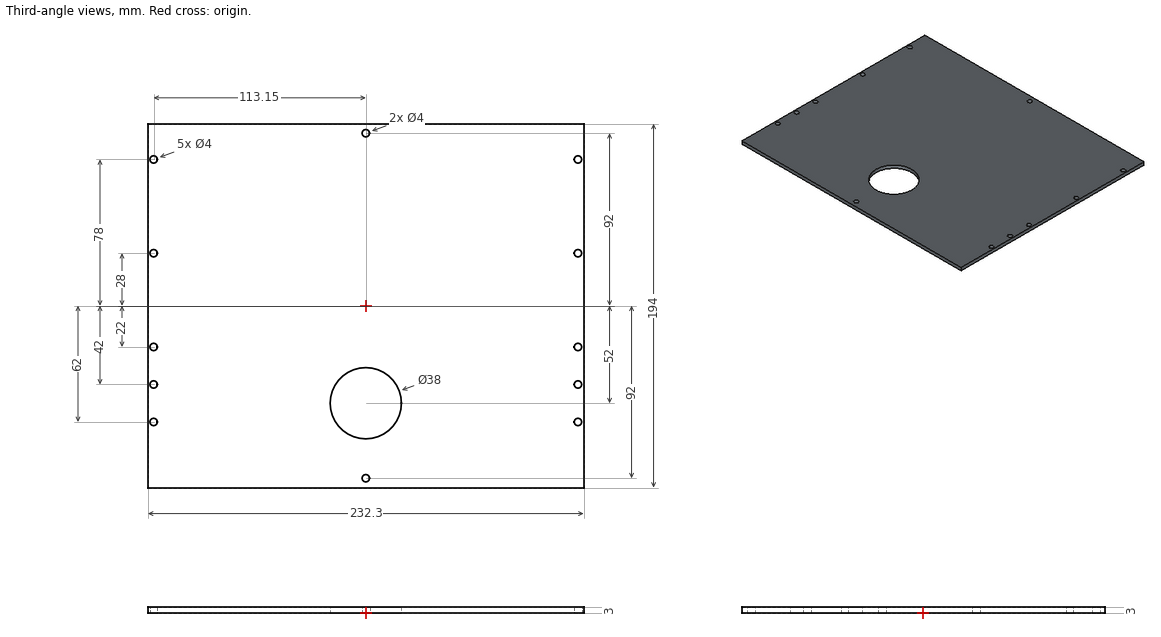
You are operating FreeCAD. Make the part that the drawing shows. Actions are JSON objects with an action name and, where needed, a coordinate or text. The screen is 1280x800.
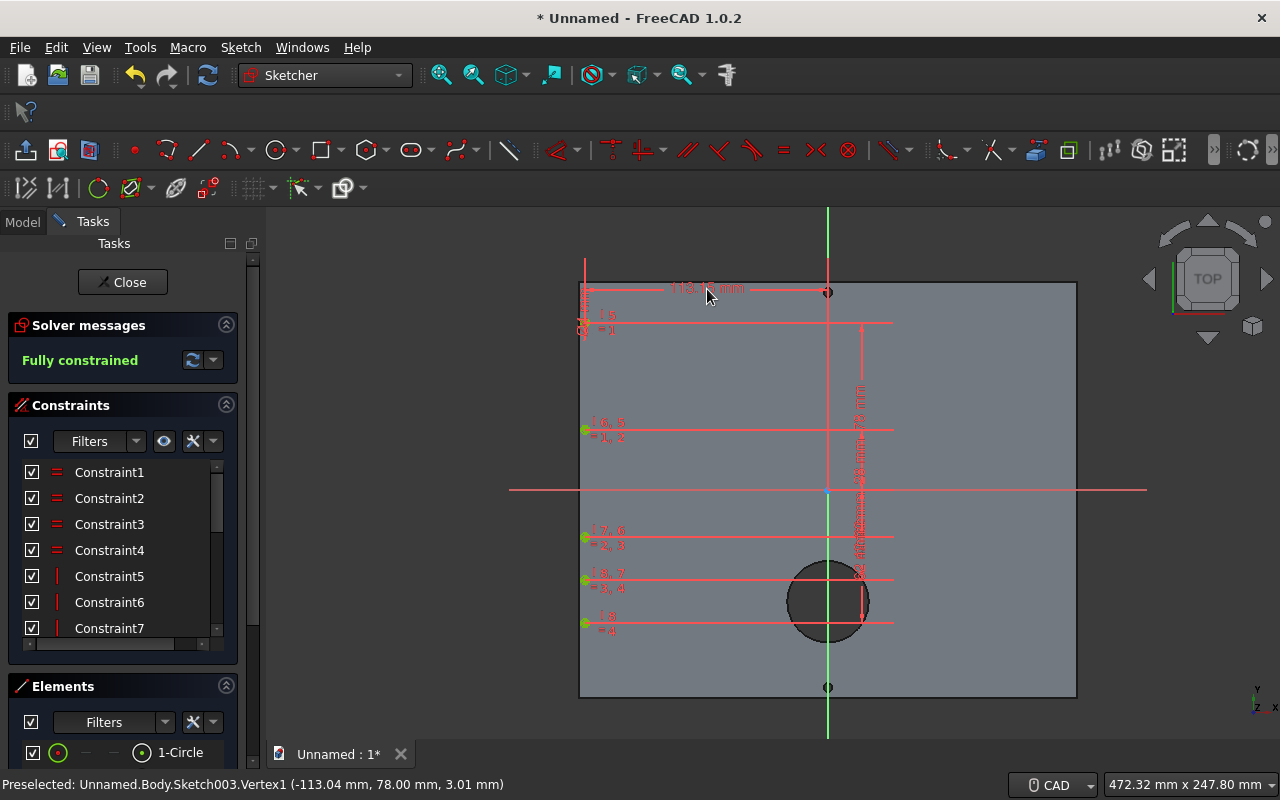
{"action": "left_click", "coordinate": [123, 282]}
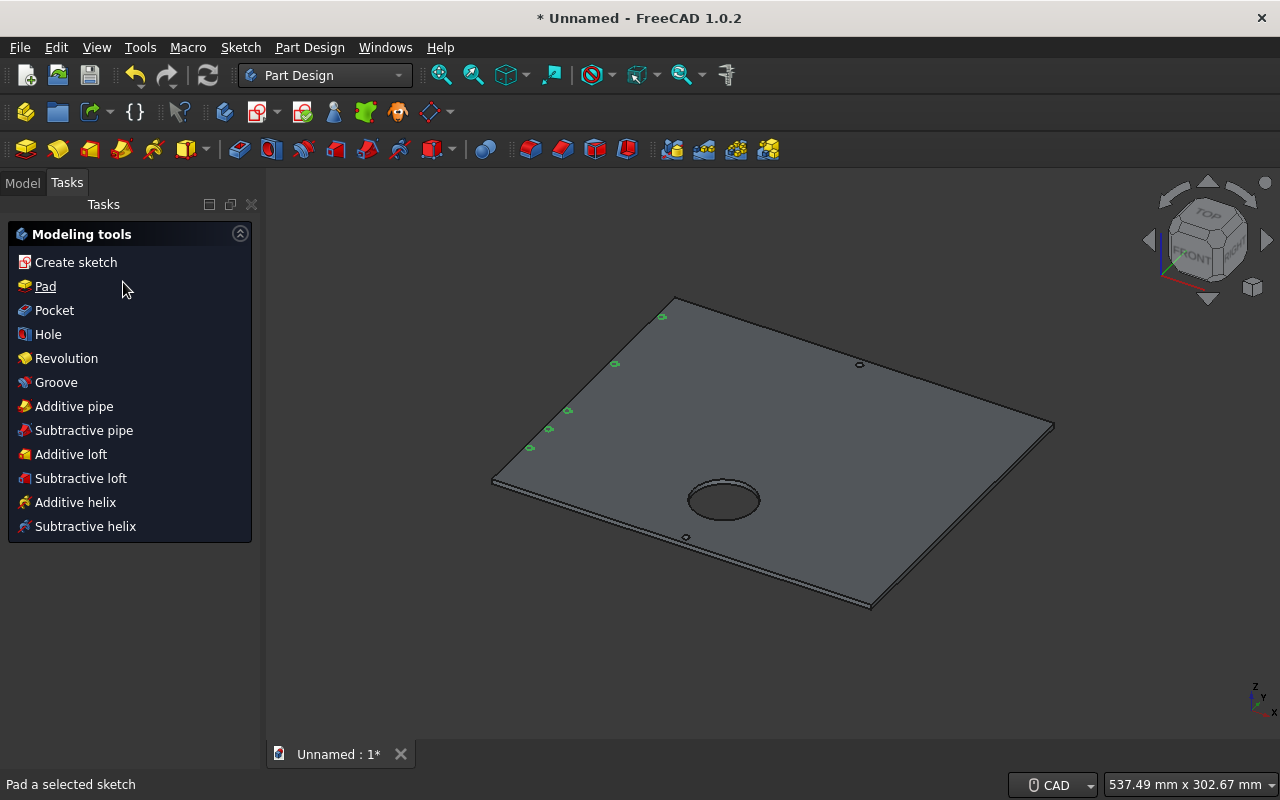
{"action": "left_click", "coordinate": [240, 150]}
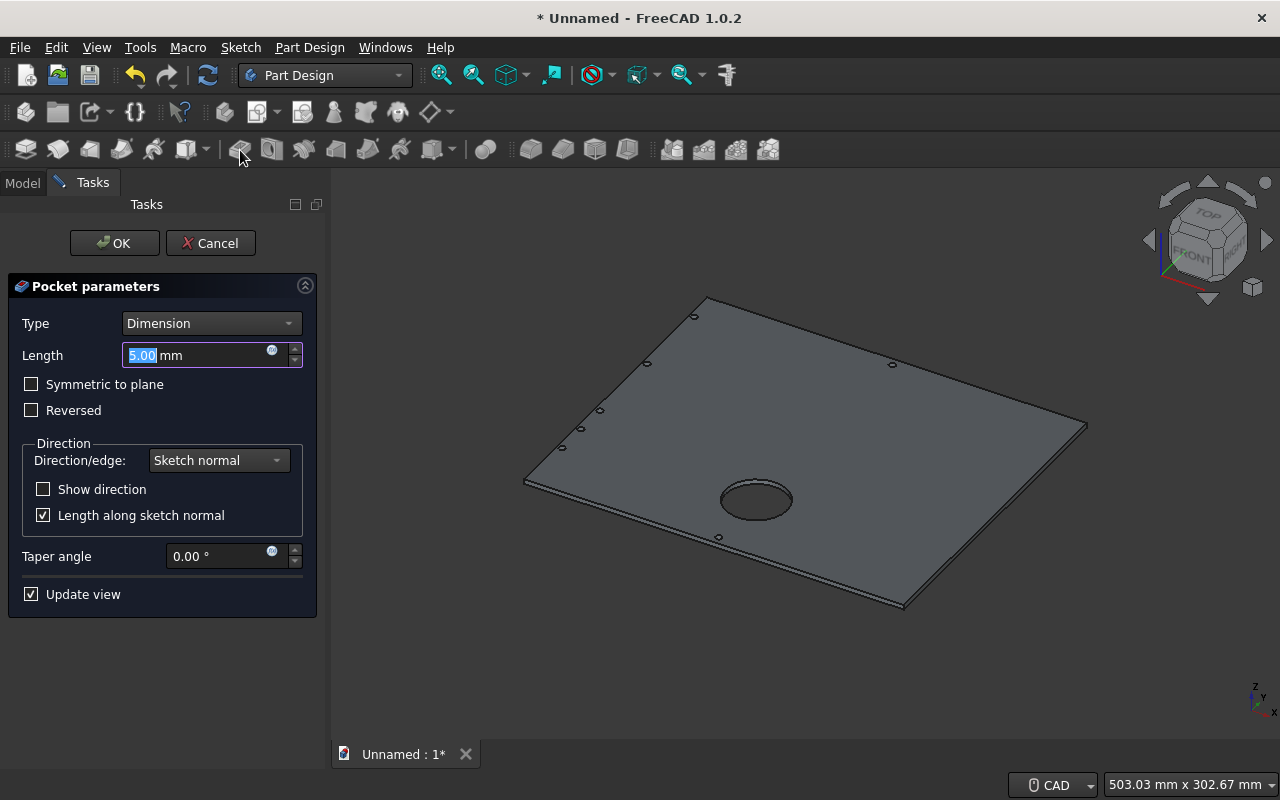
{"action": "left_click", "coordinate": [212, 324]}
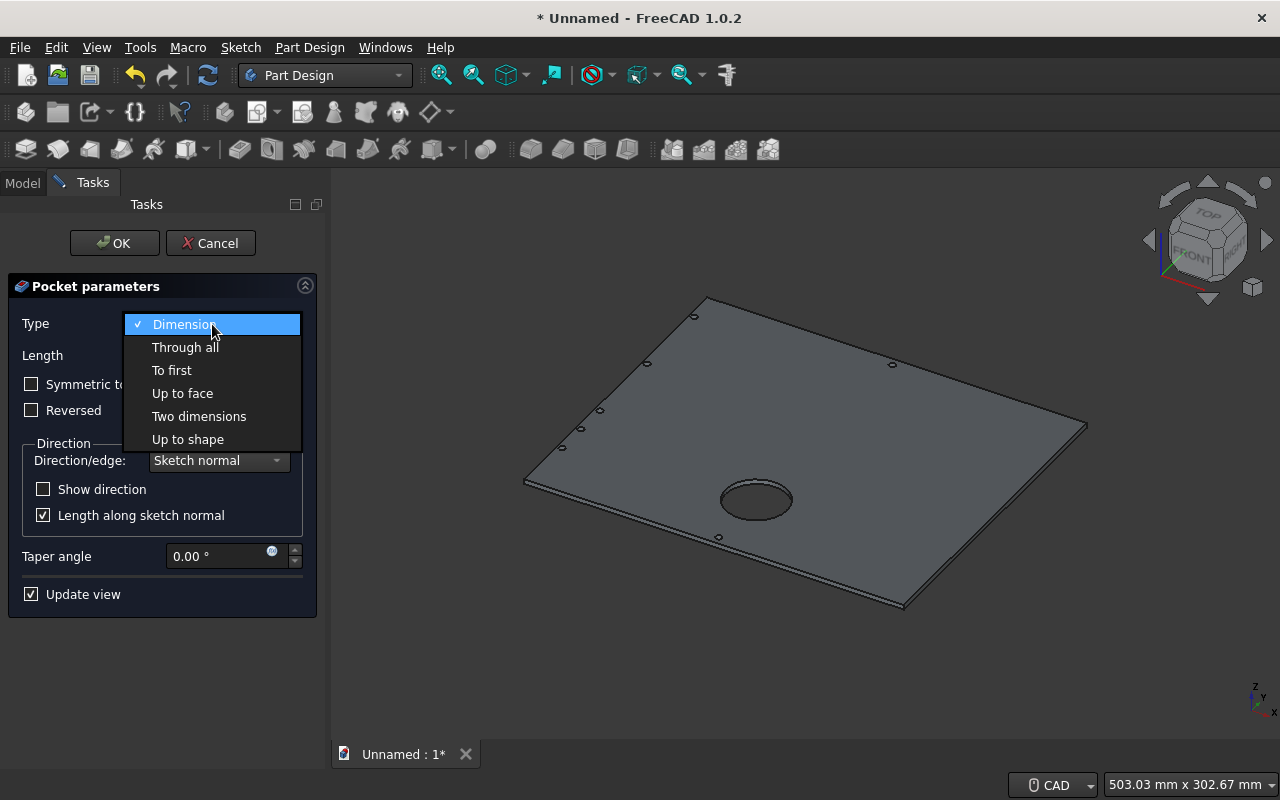
{"action": "left_click", "coordinate": [212, 348]}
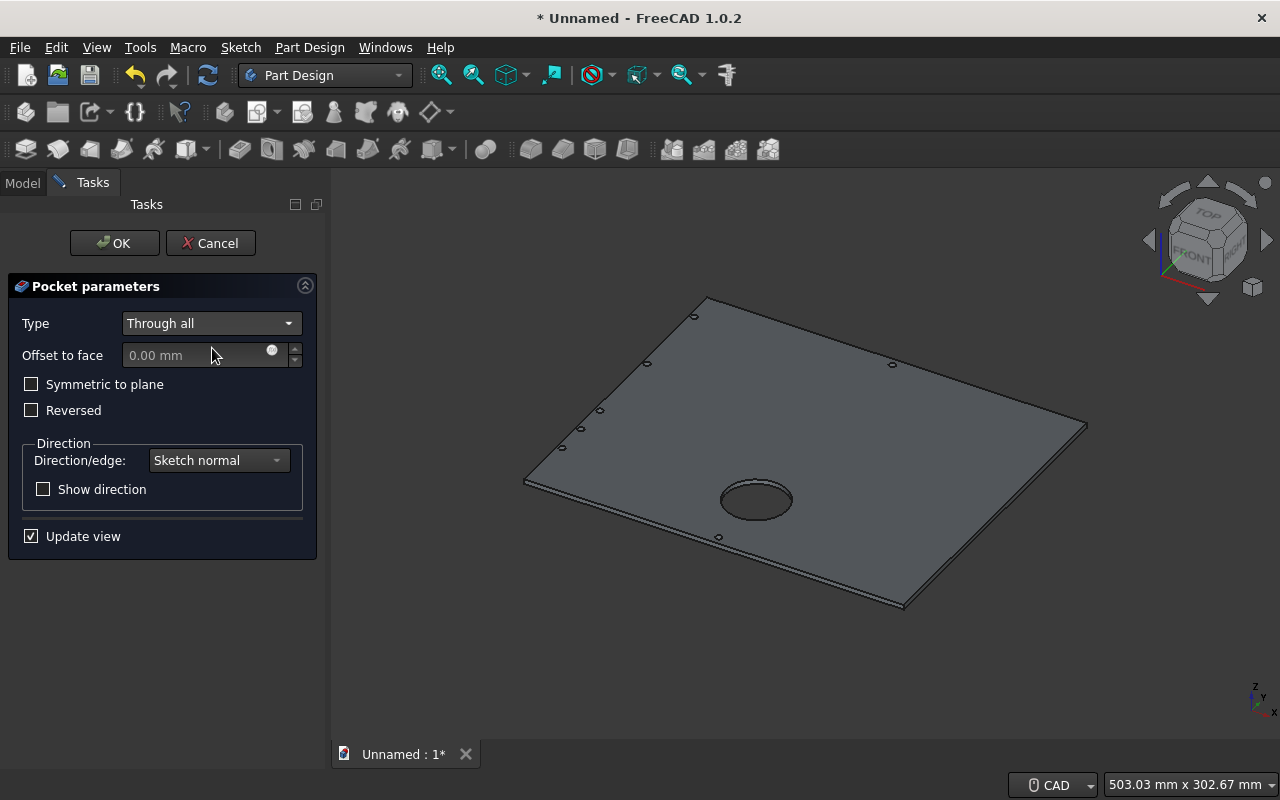
{"action": "left_click", "coordinate": [115, 243]}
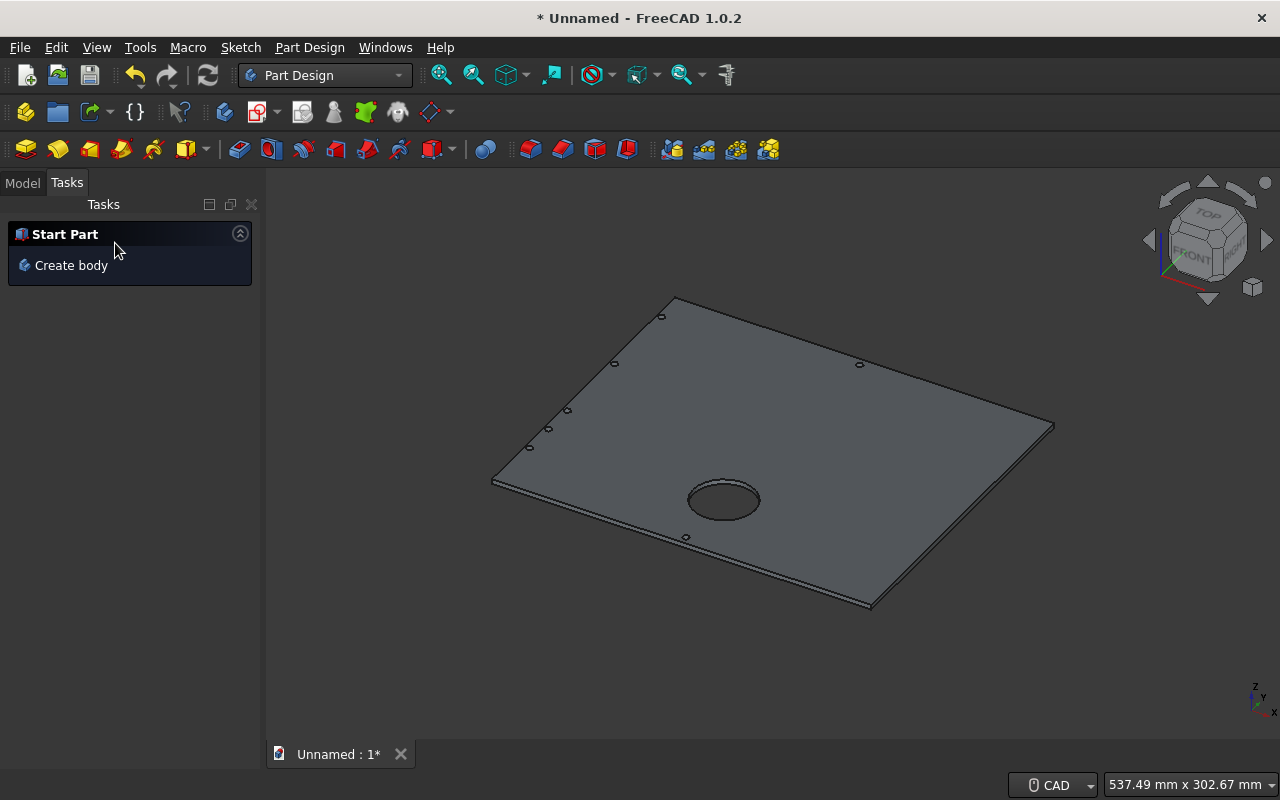
{"action": "left_click", "coordinate": [23, 182]}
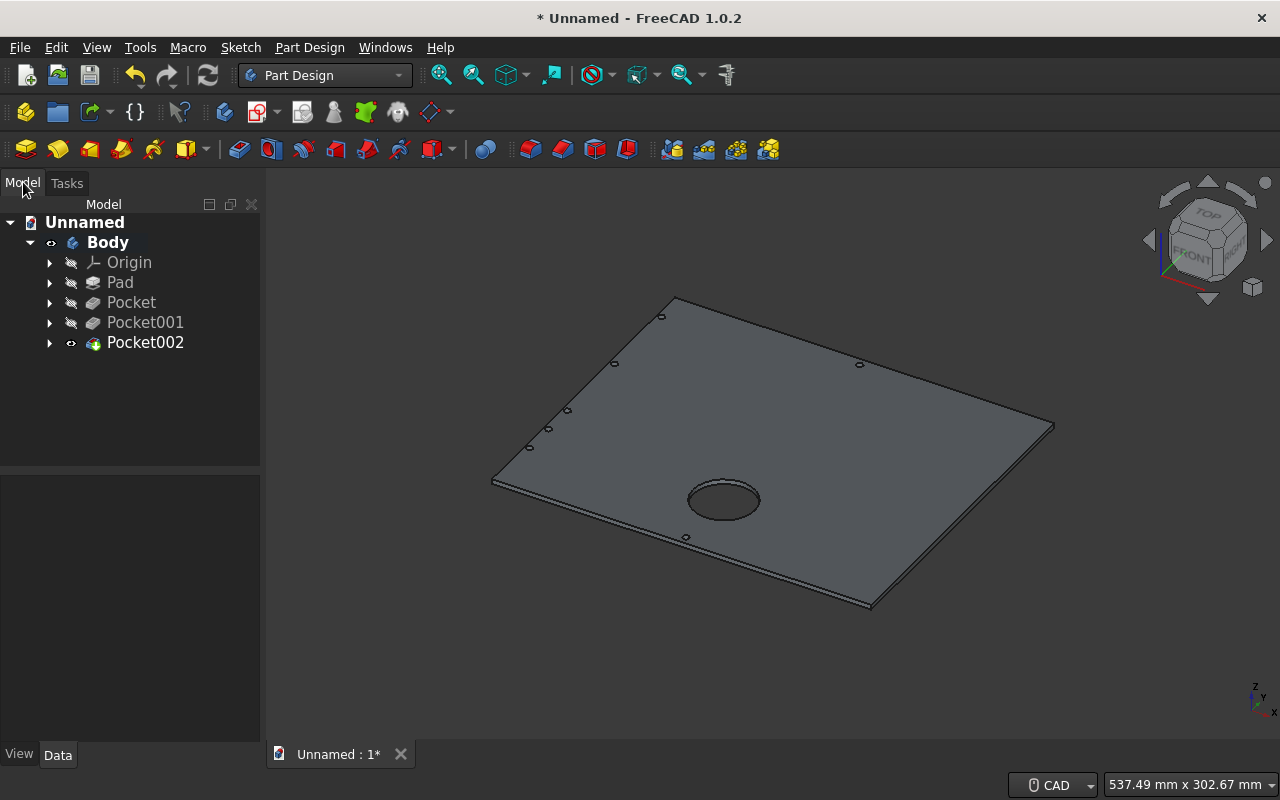
{"action": "left_click", "coordinate": [116, 343]}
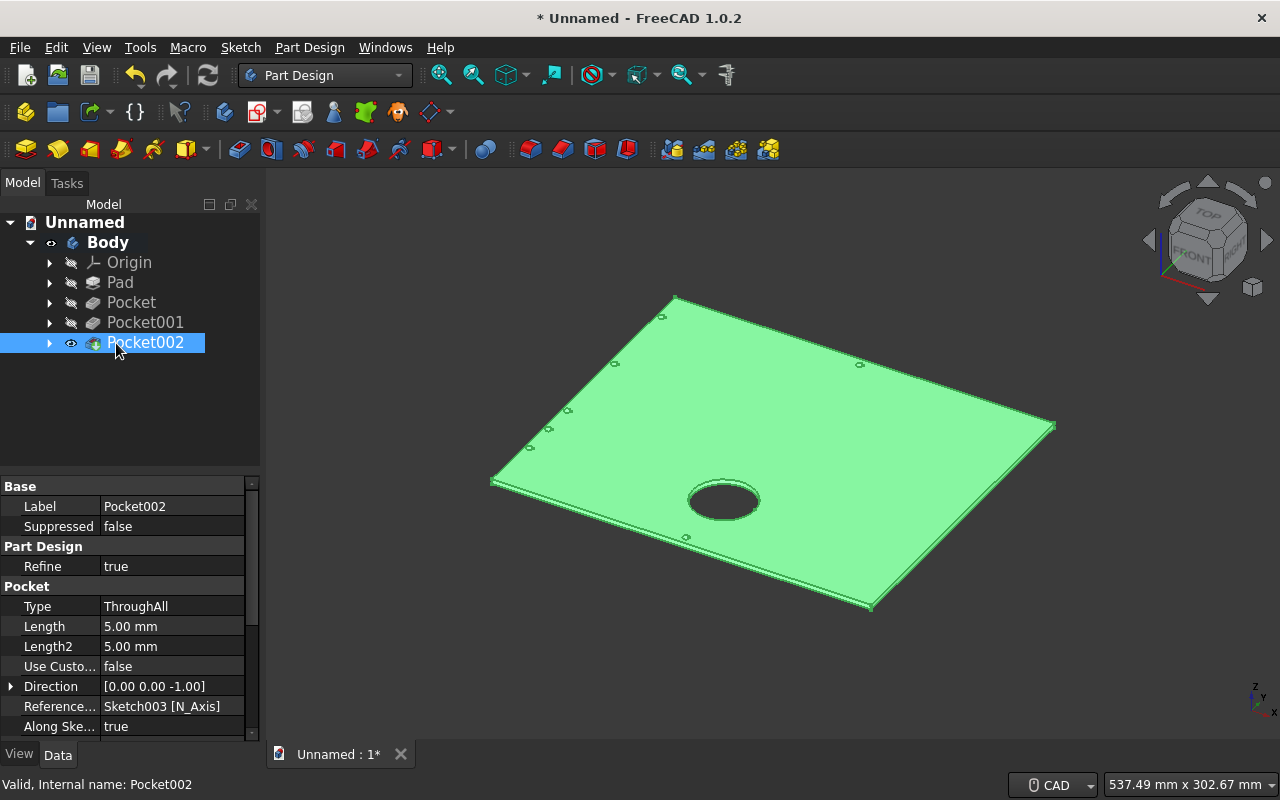
{"action": "left_click", "coordinate": [672, 150]}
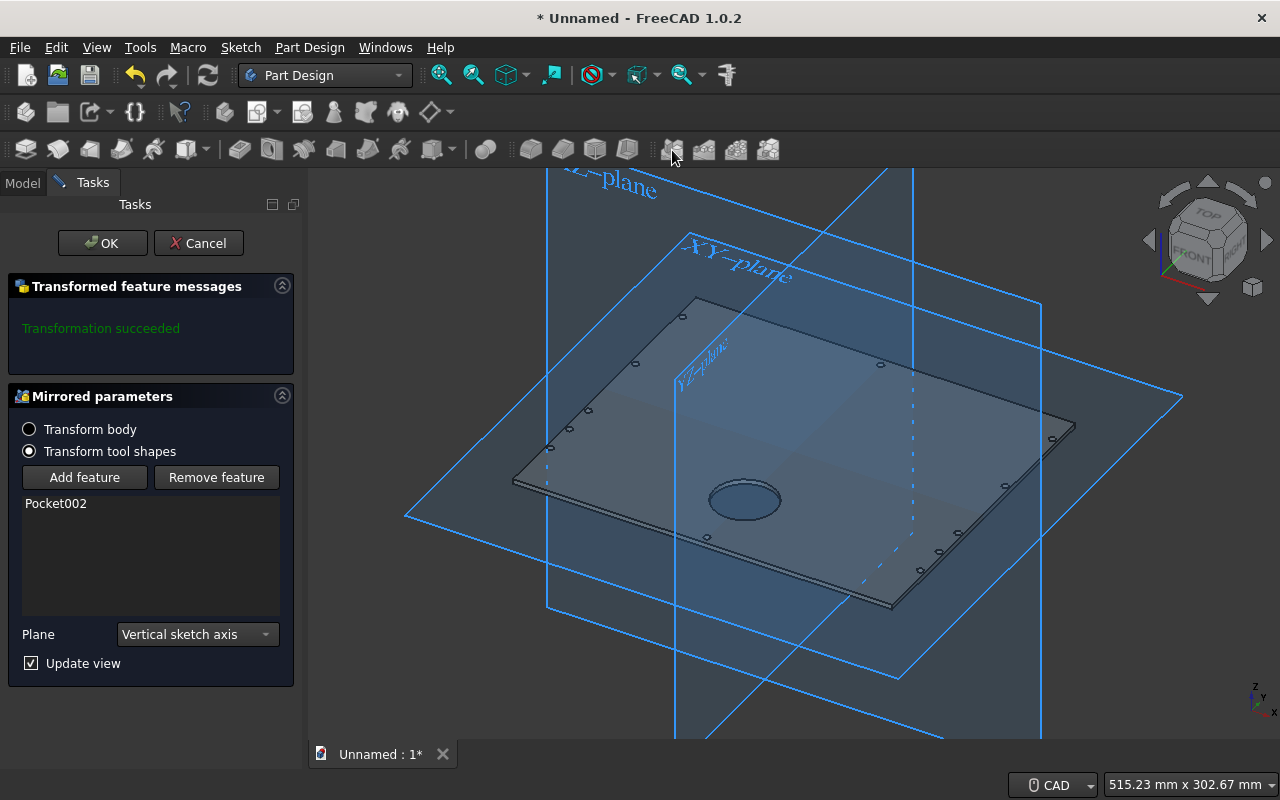
{"action": "left_click", "coordinate": [198, 634]}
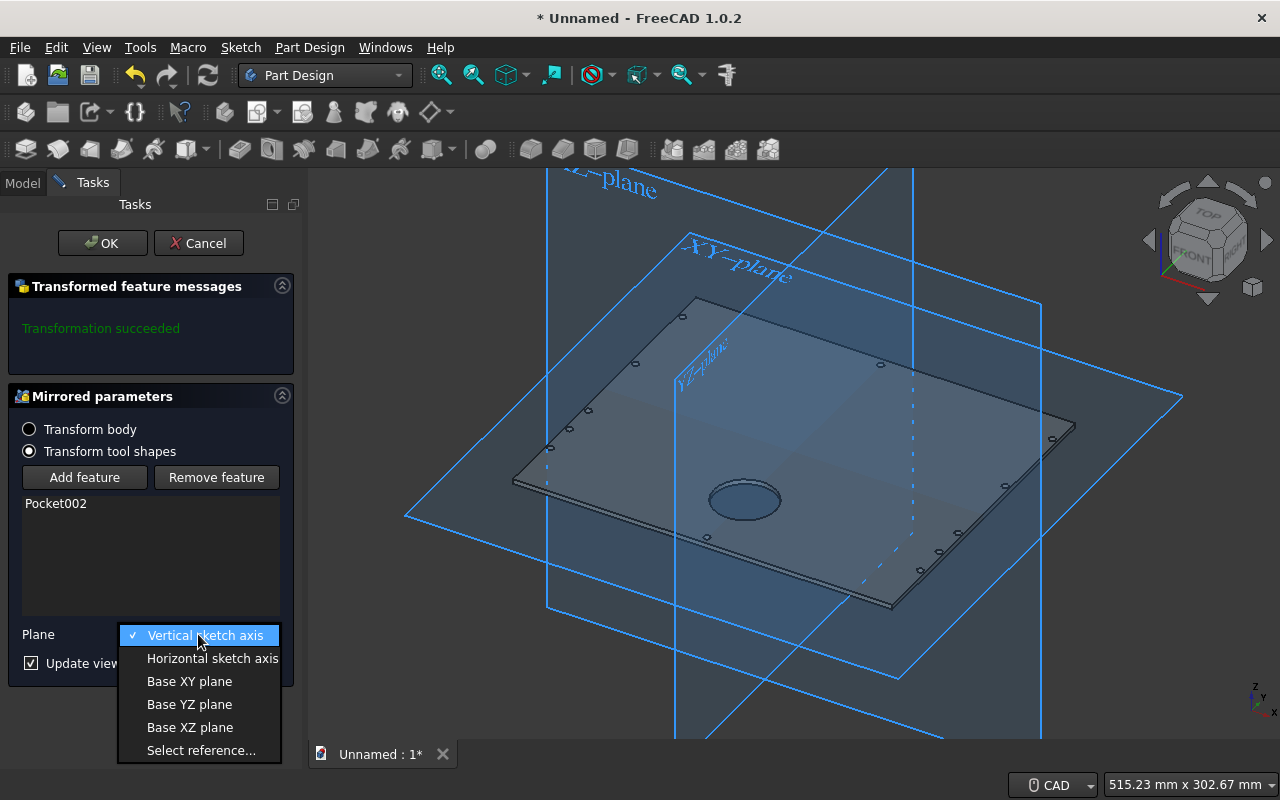
{"action": "left_click", "coordinate": [198, 704]}